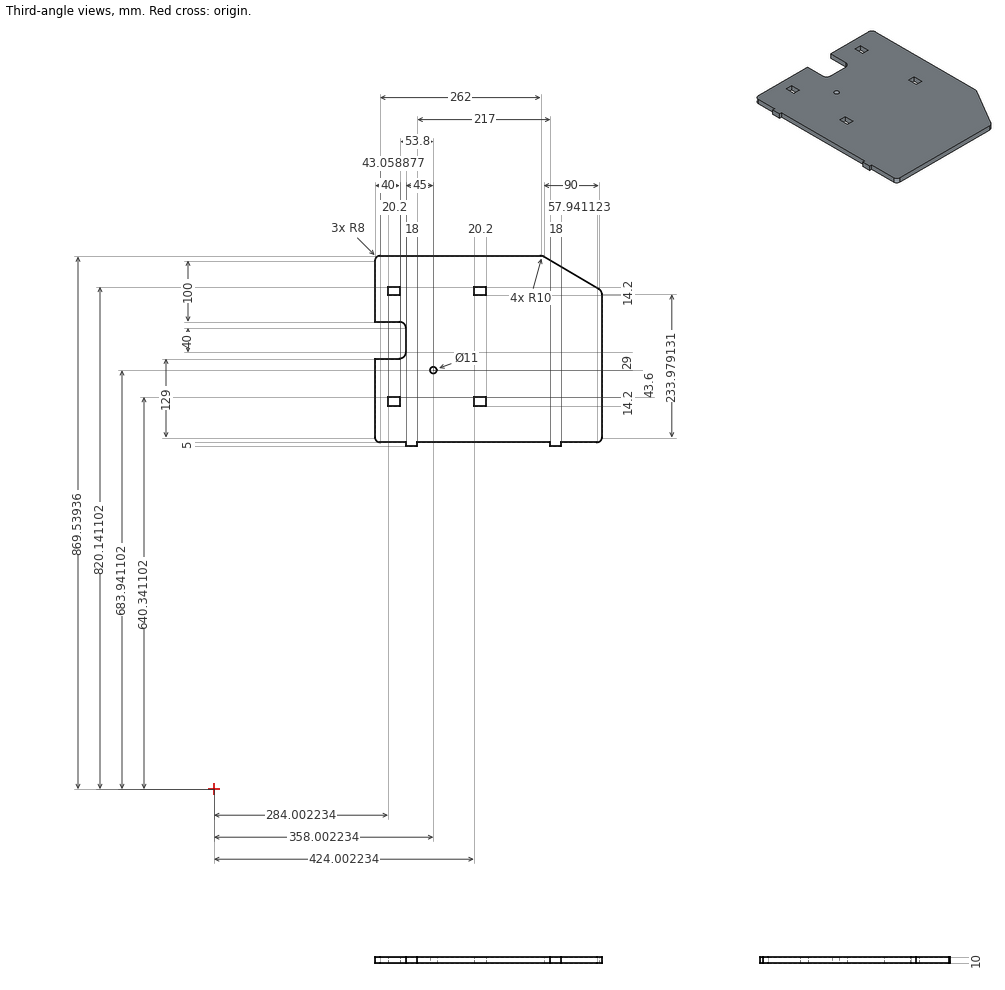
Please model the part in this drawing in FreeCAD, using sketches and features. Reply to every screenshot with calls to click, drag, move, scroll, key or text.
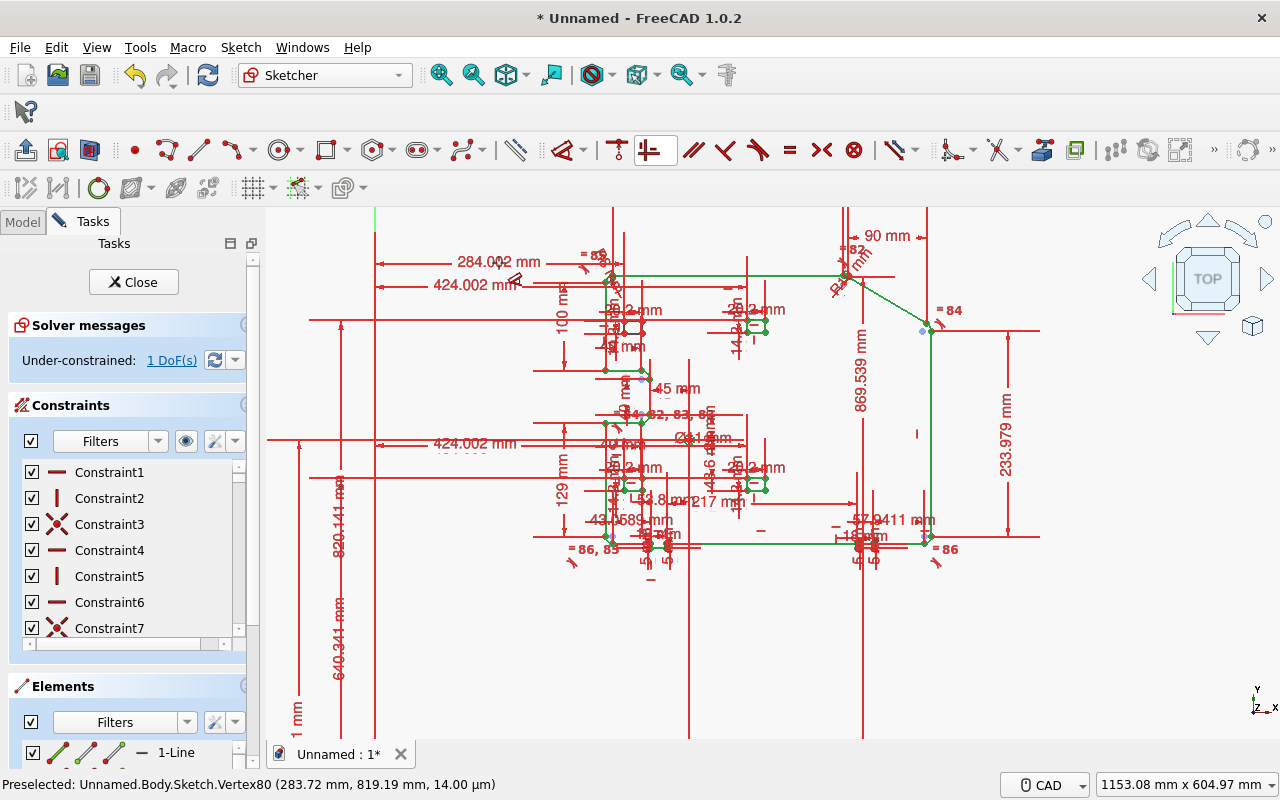
click(624, 321)
click(341, 426)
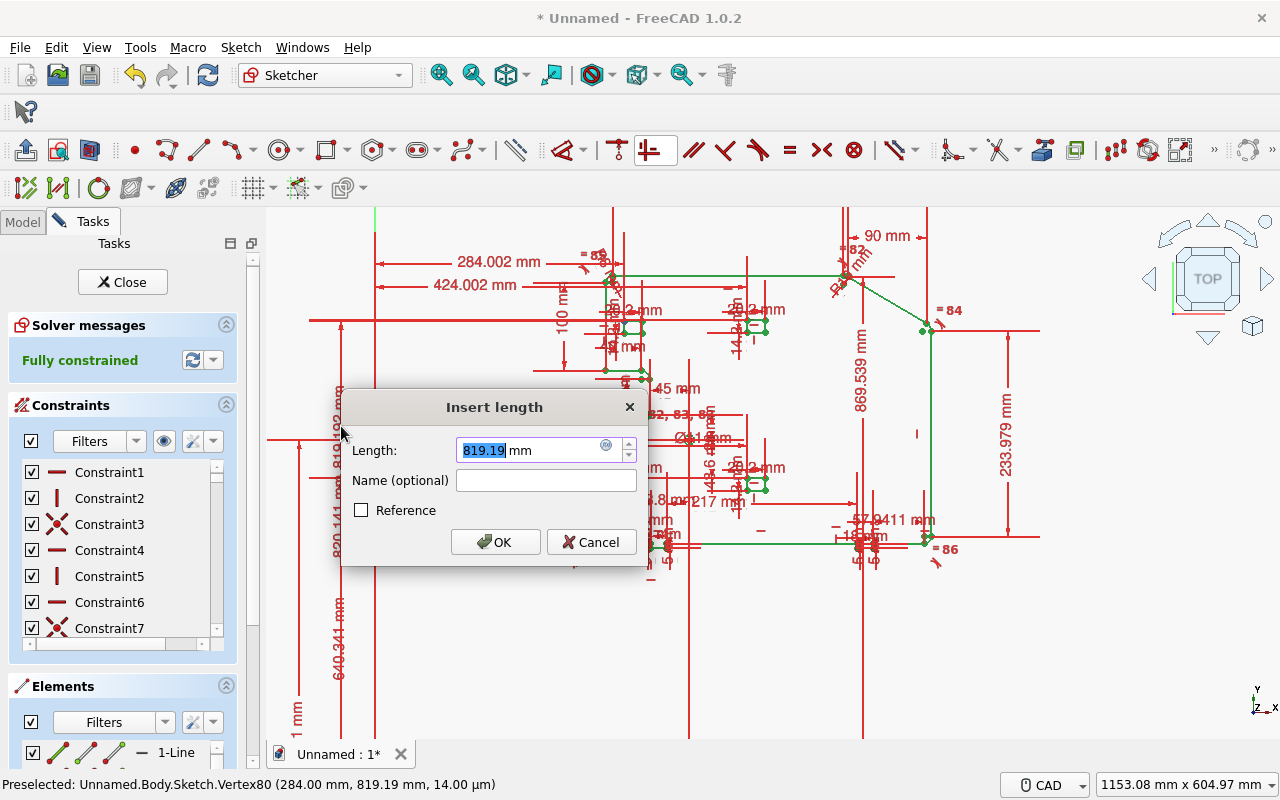
text(820.141102)
key(Return)
key(Escape)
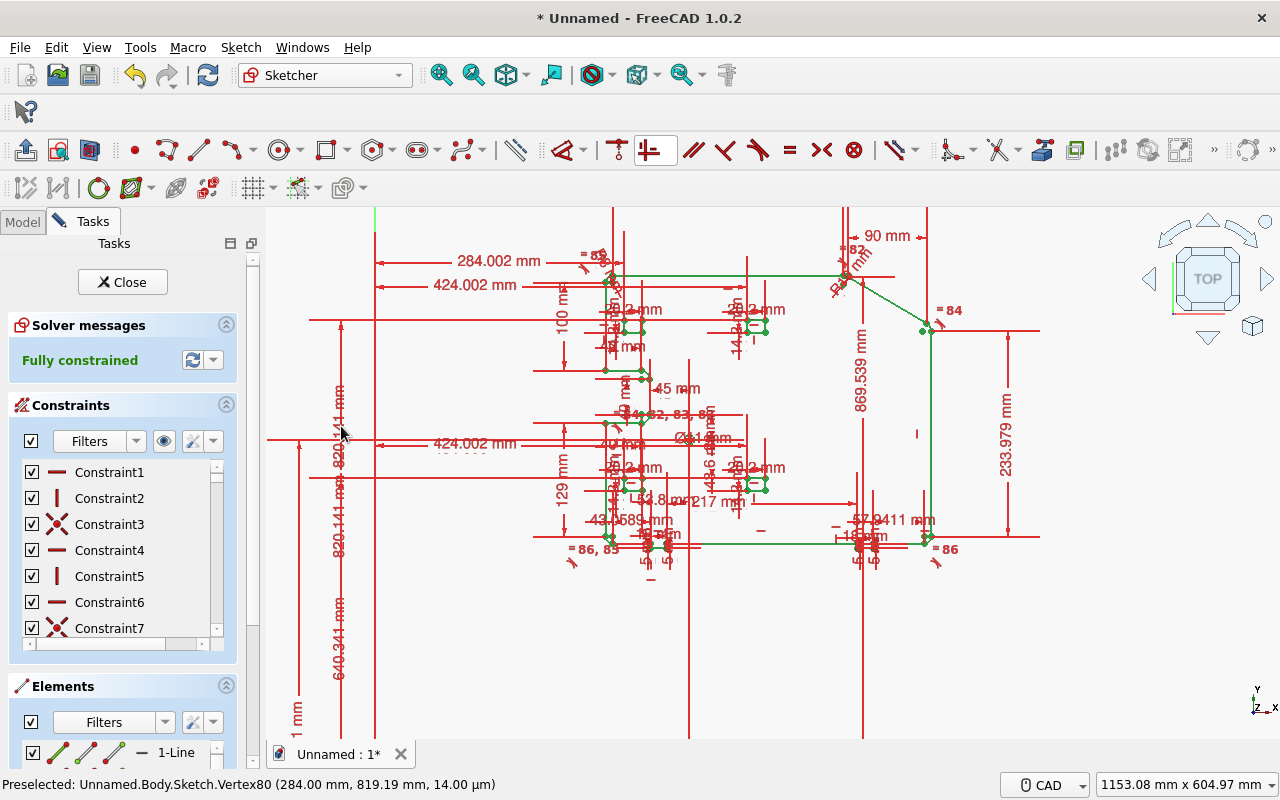
click(123, 282)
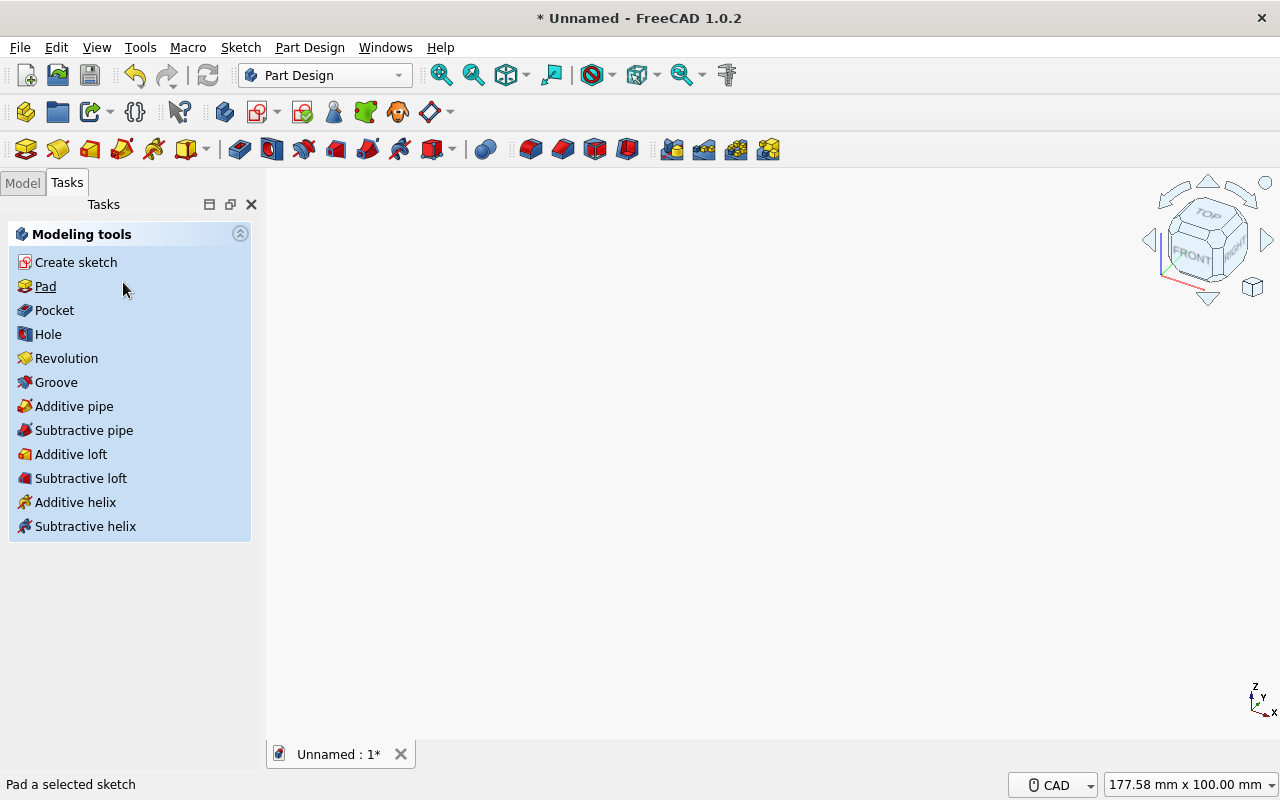
click(26, 150)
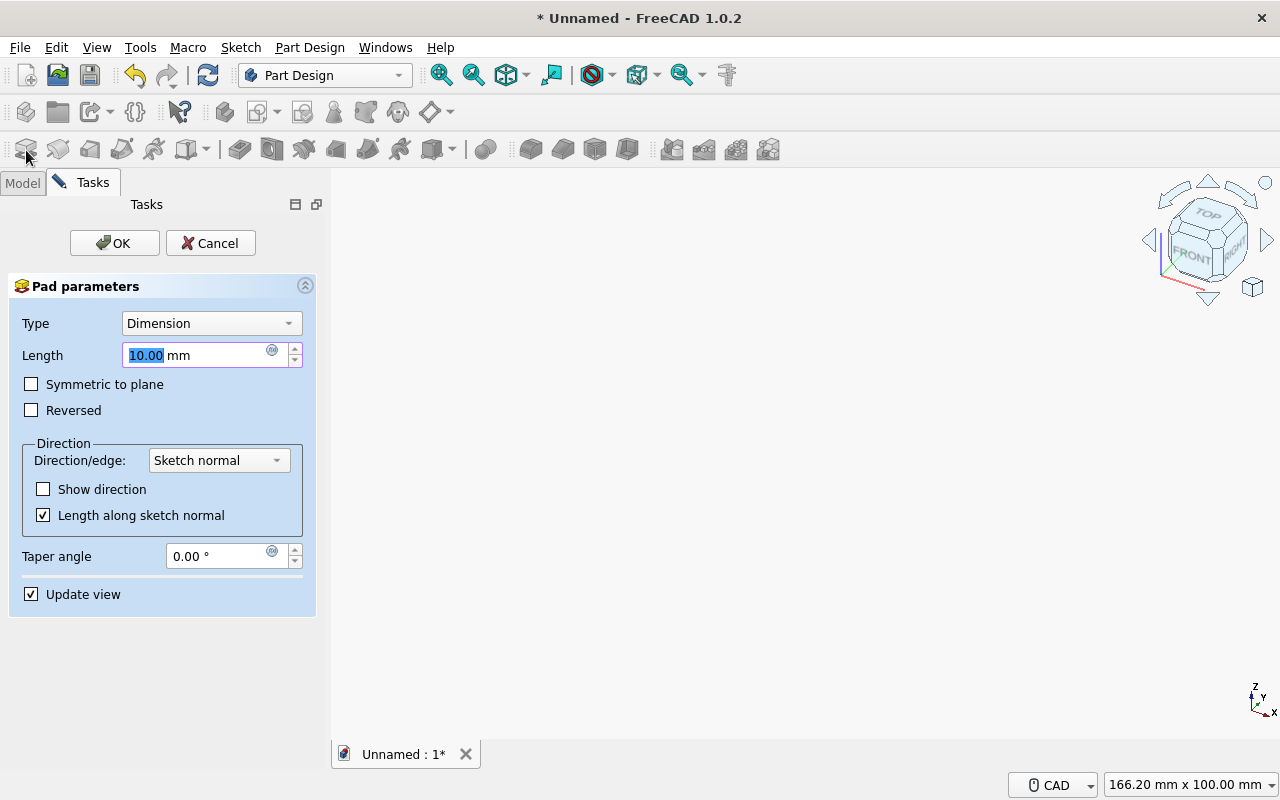
text(10)
key(Tab)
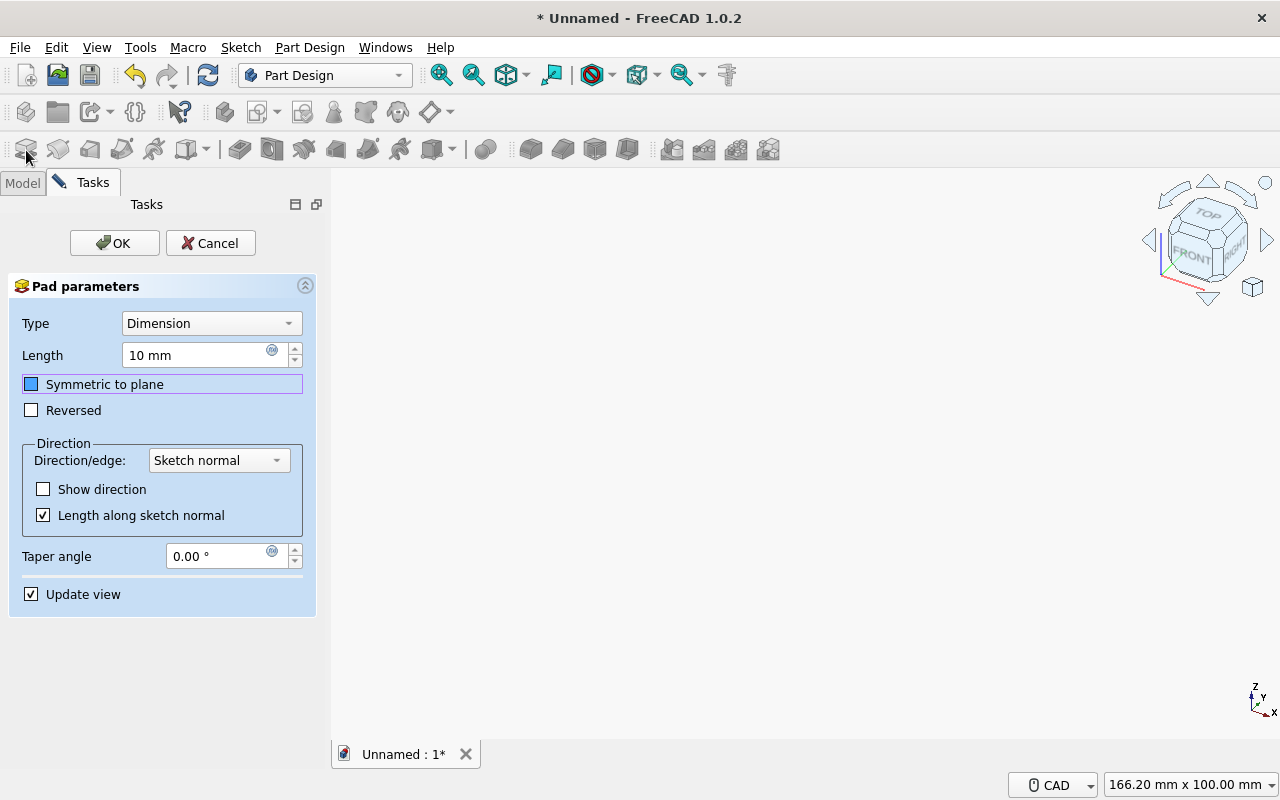
click(115, 243)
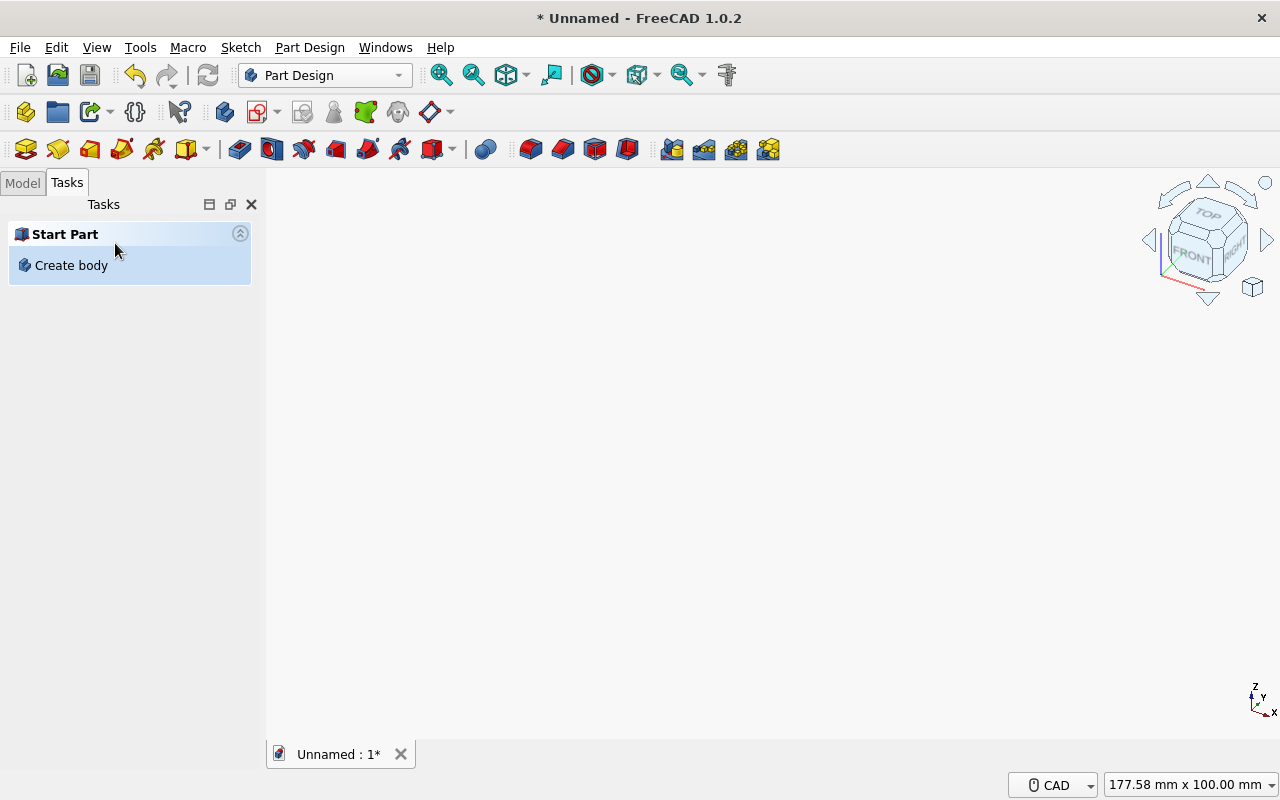
key(0)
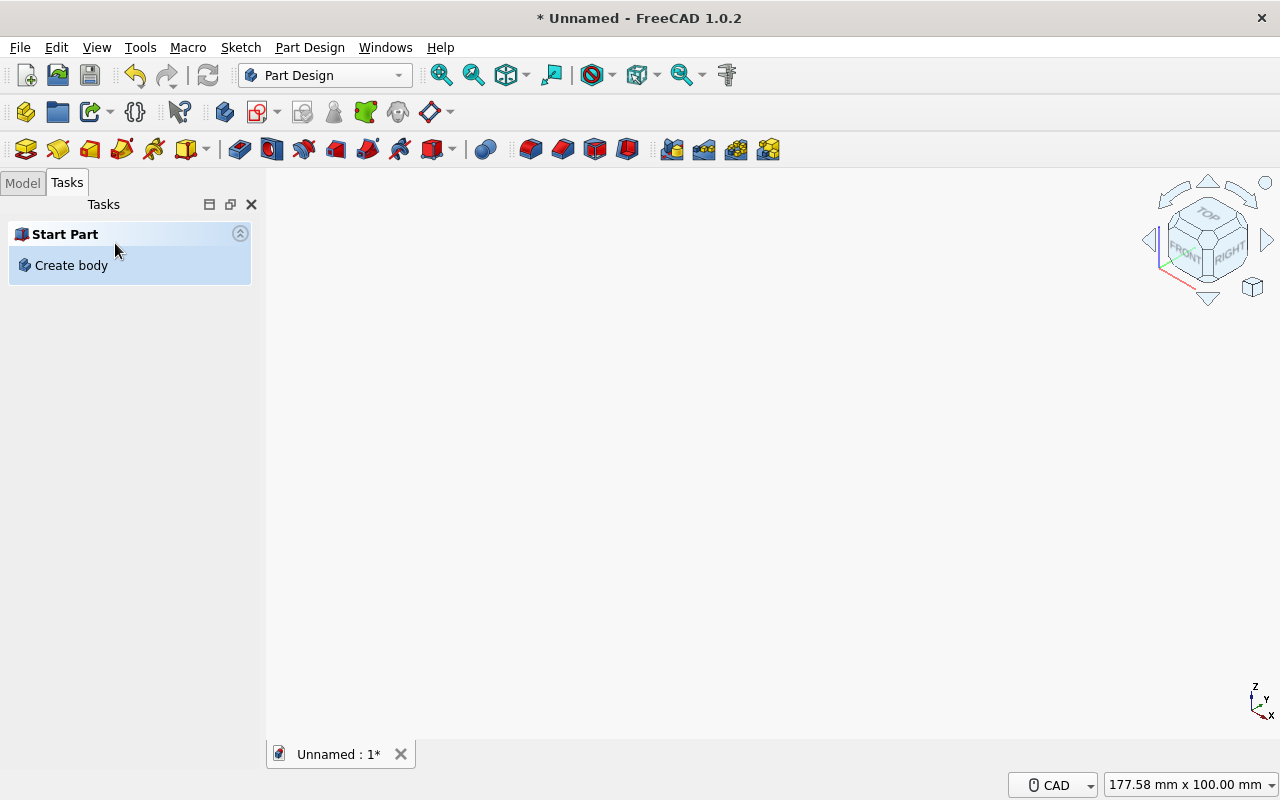
click(442, 76)